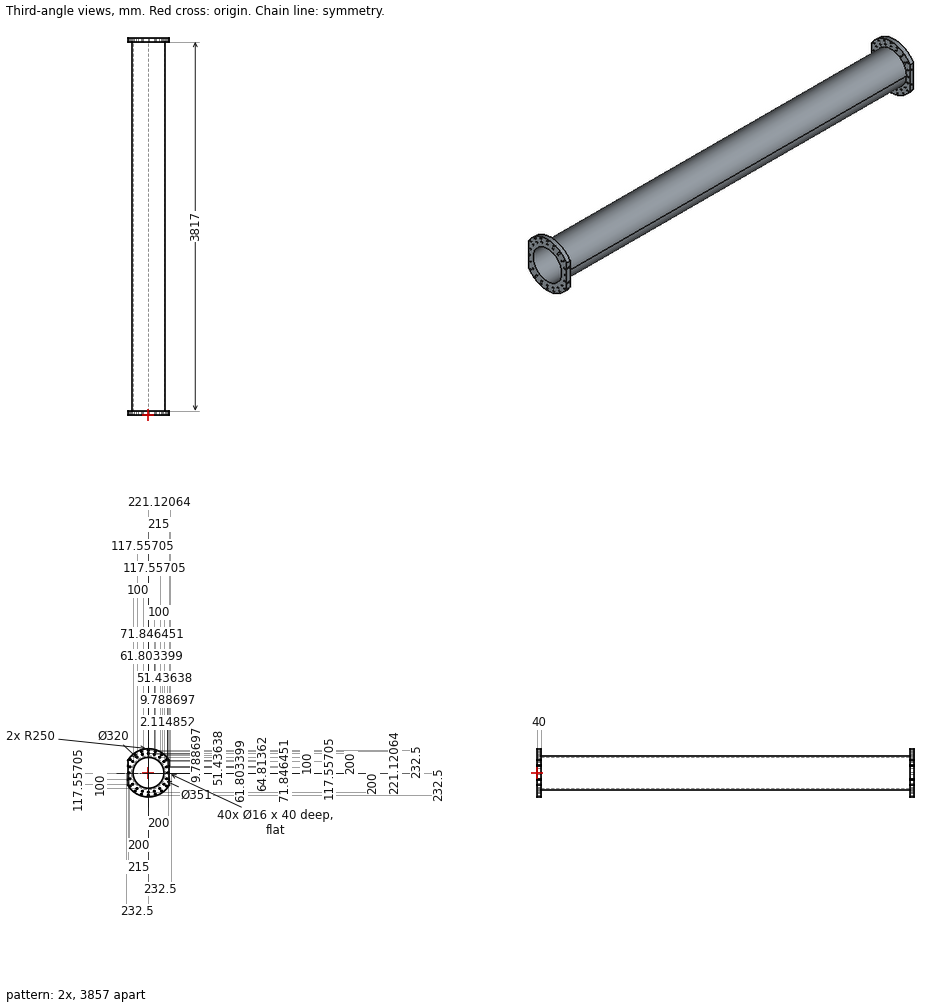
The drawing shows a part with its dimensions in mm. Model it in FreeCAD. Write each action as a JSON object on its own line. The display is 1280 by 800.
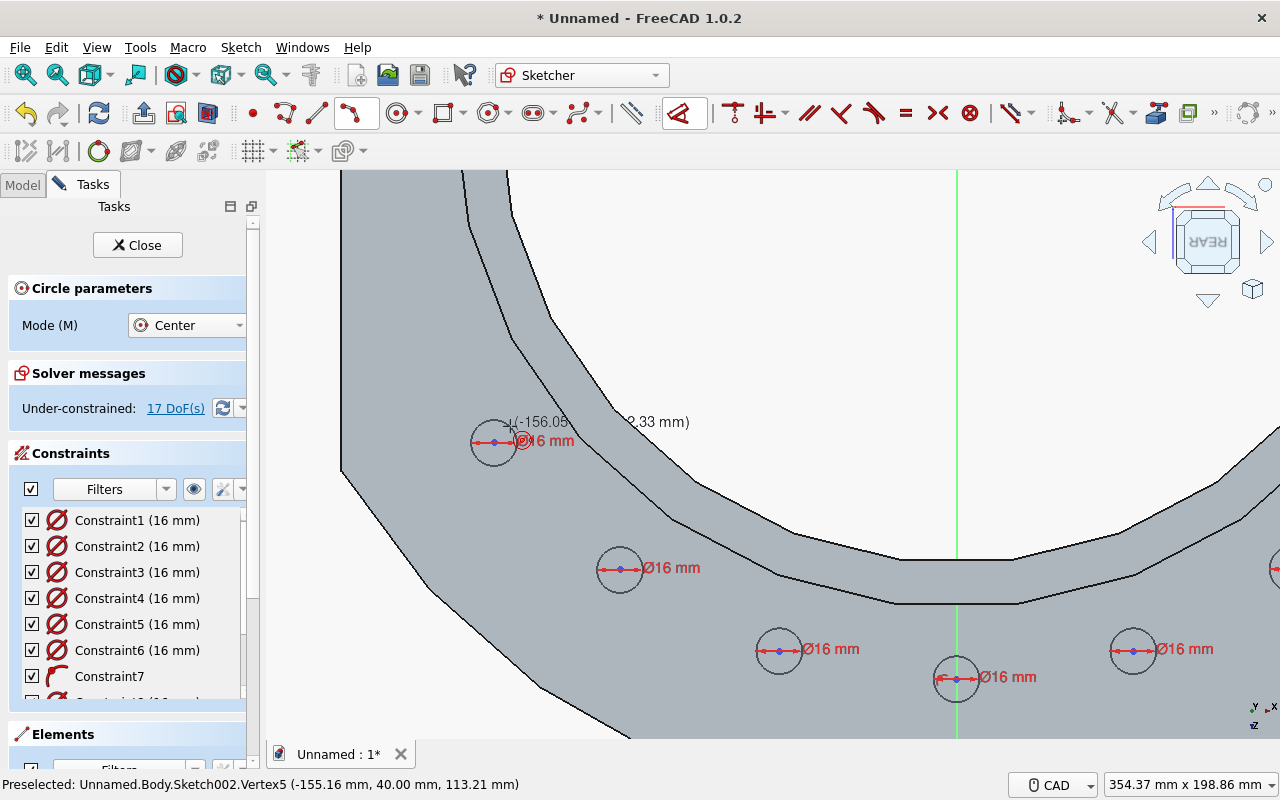
{"action": "left_click", "coordinate": [412, 282]}
{"action": "mouse_move", "coordinate": [428, 266]}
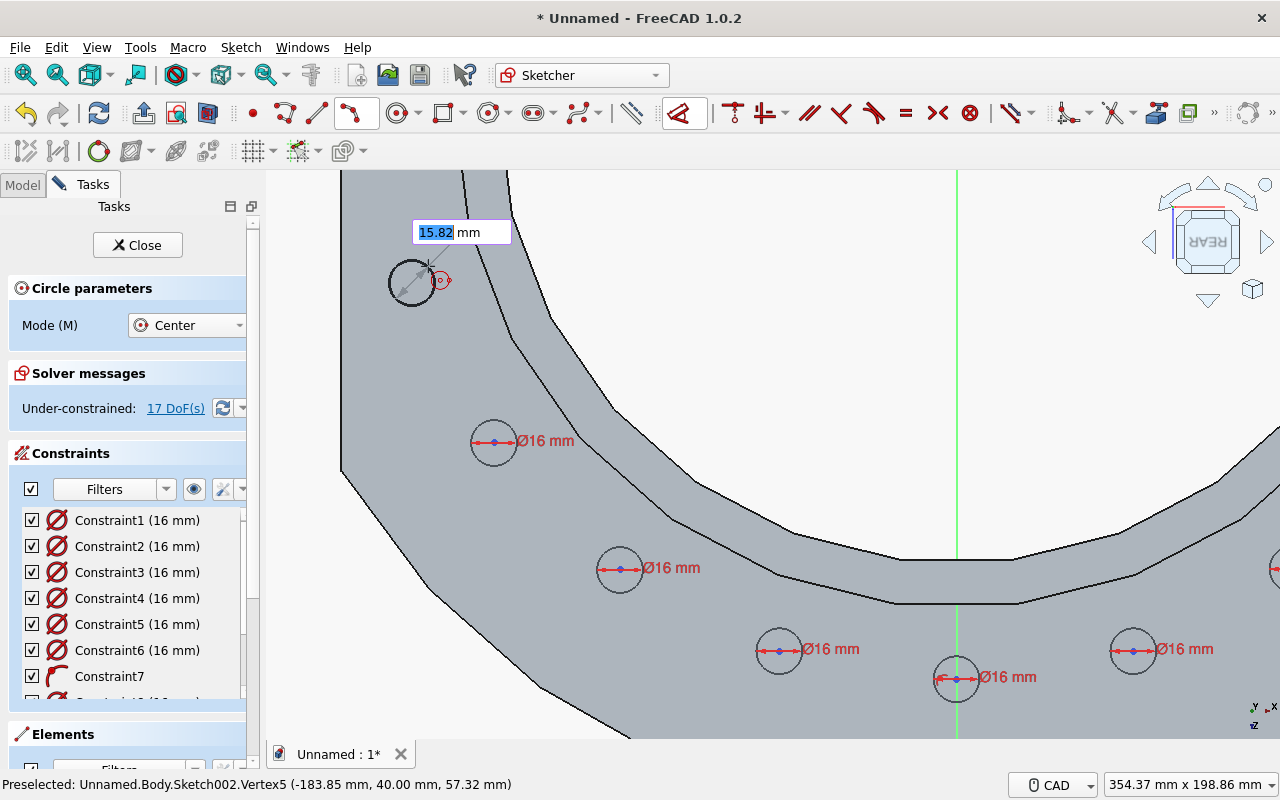
{"action": "type", "text": "16"}
{"action": "key", "text": "Return"}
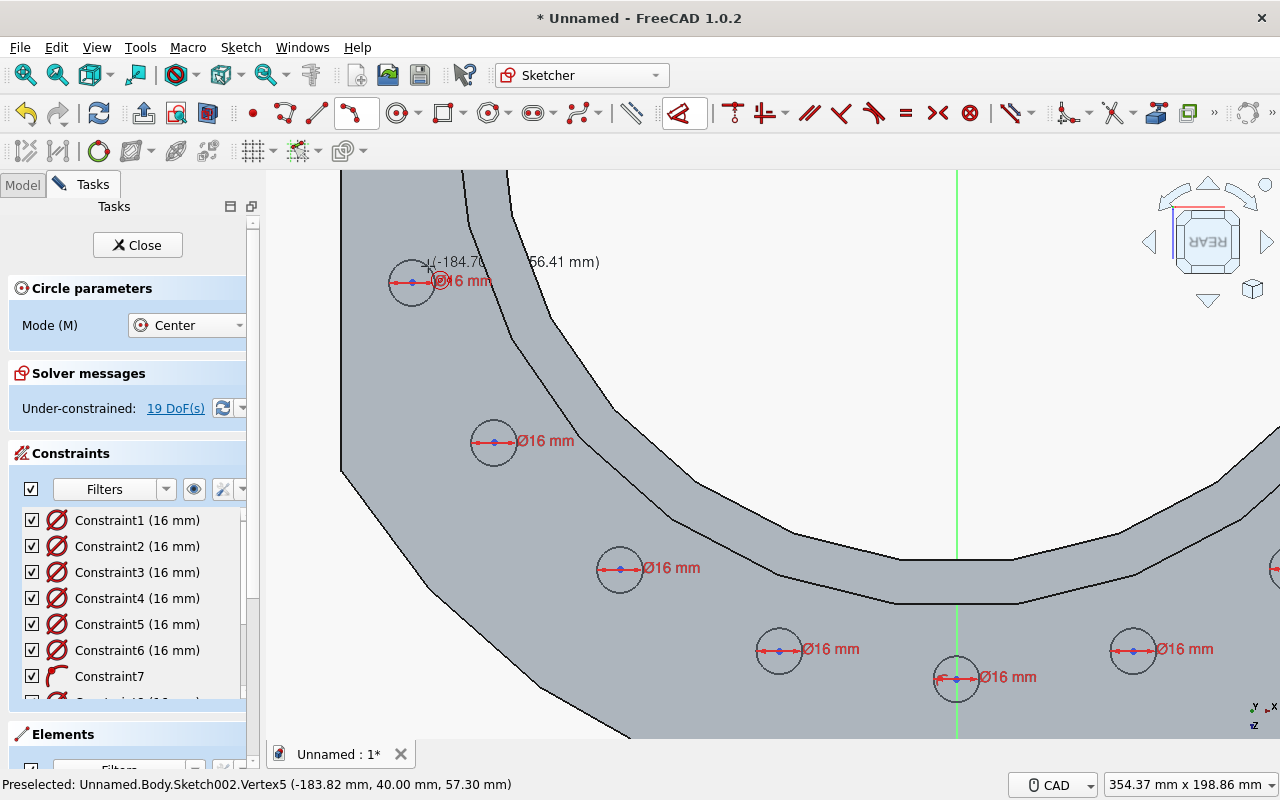
{"action": "scroll", "coordinate": [622, 569], "scroll_direction": "down", "scroll_amount": 7}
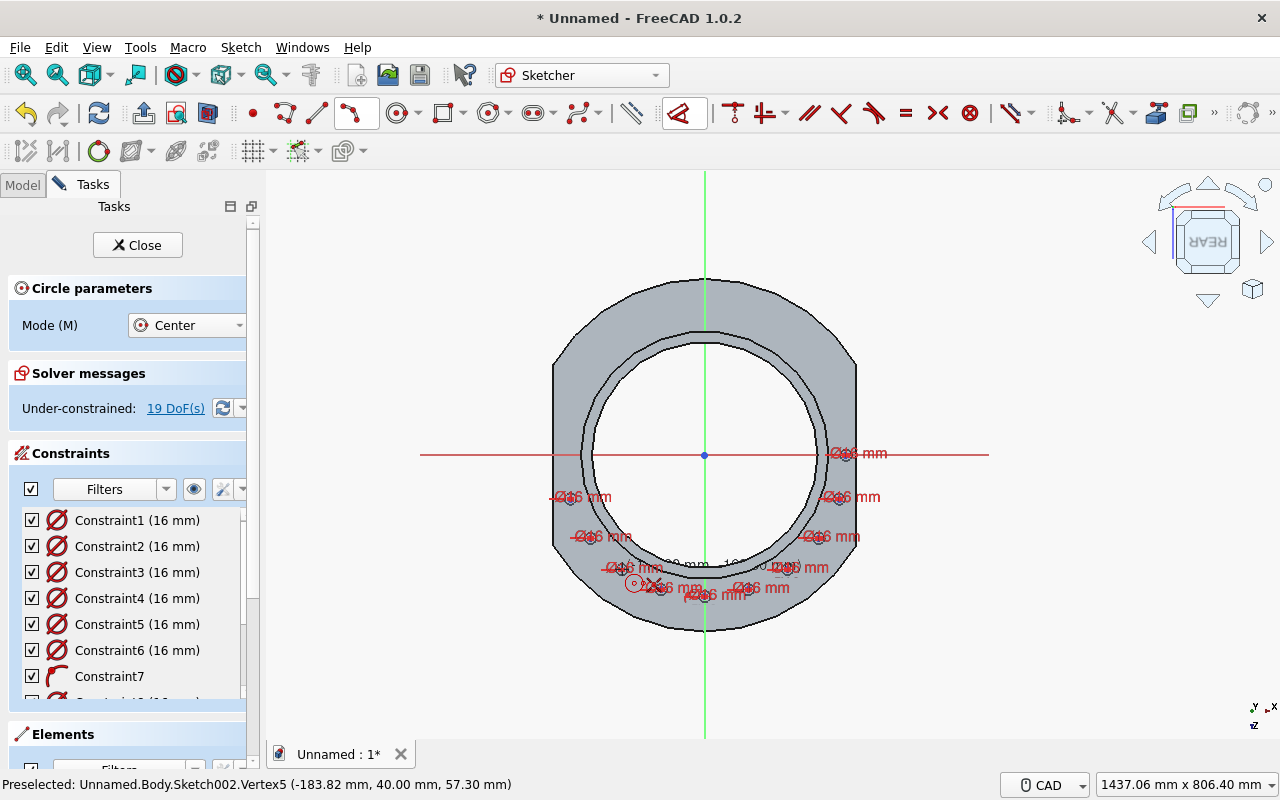
{"action": "scroll", "coordinate": [564, 455], "scroll_direction": "up", "scroll_amount": 7}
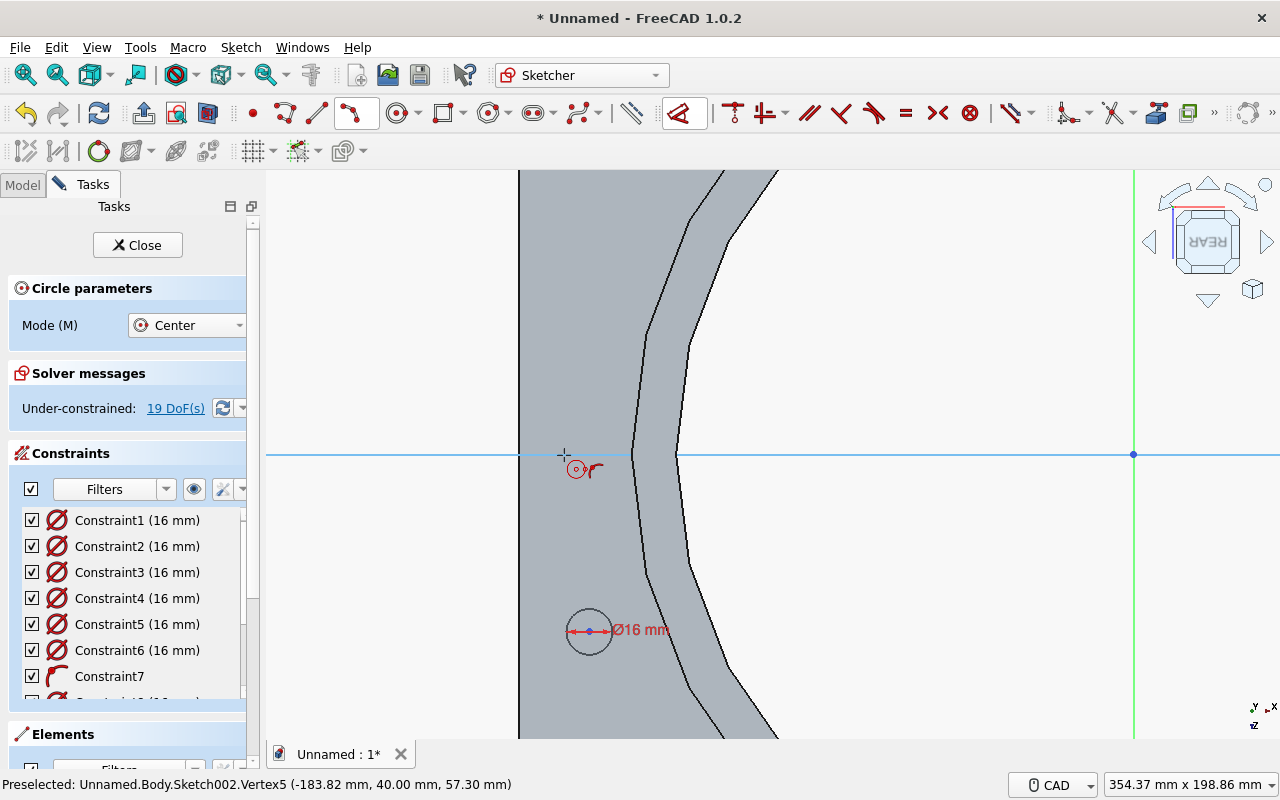
{"action": "left_click", "coordinate": [562, 455]}
{"action": "mouse_move", "coordinate": [578, 438]}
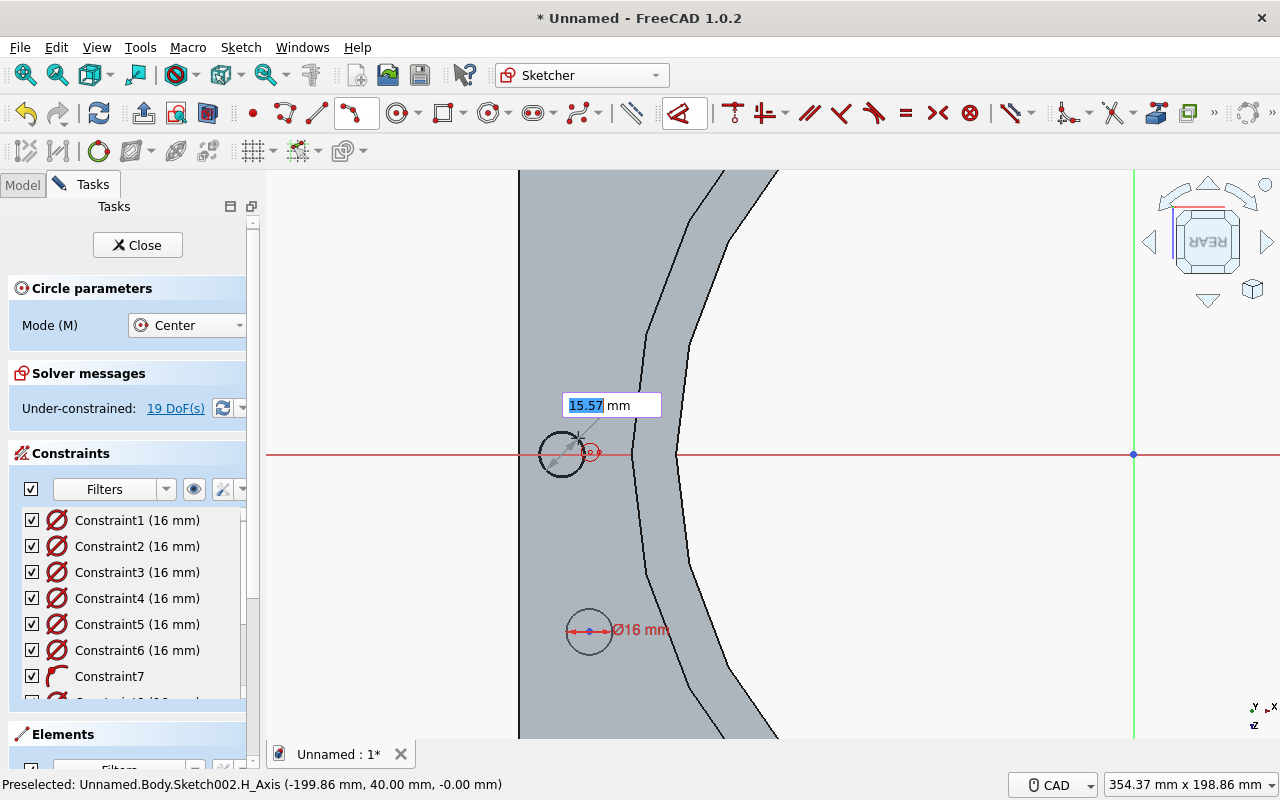
{"action": "type", "text": "16"}
{"action": "key", "text": "Return"}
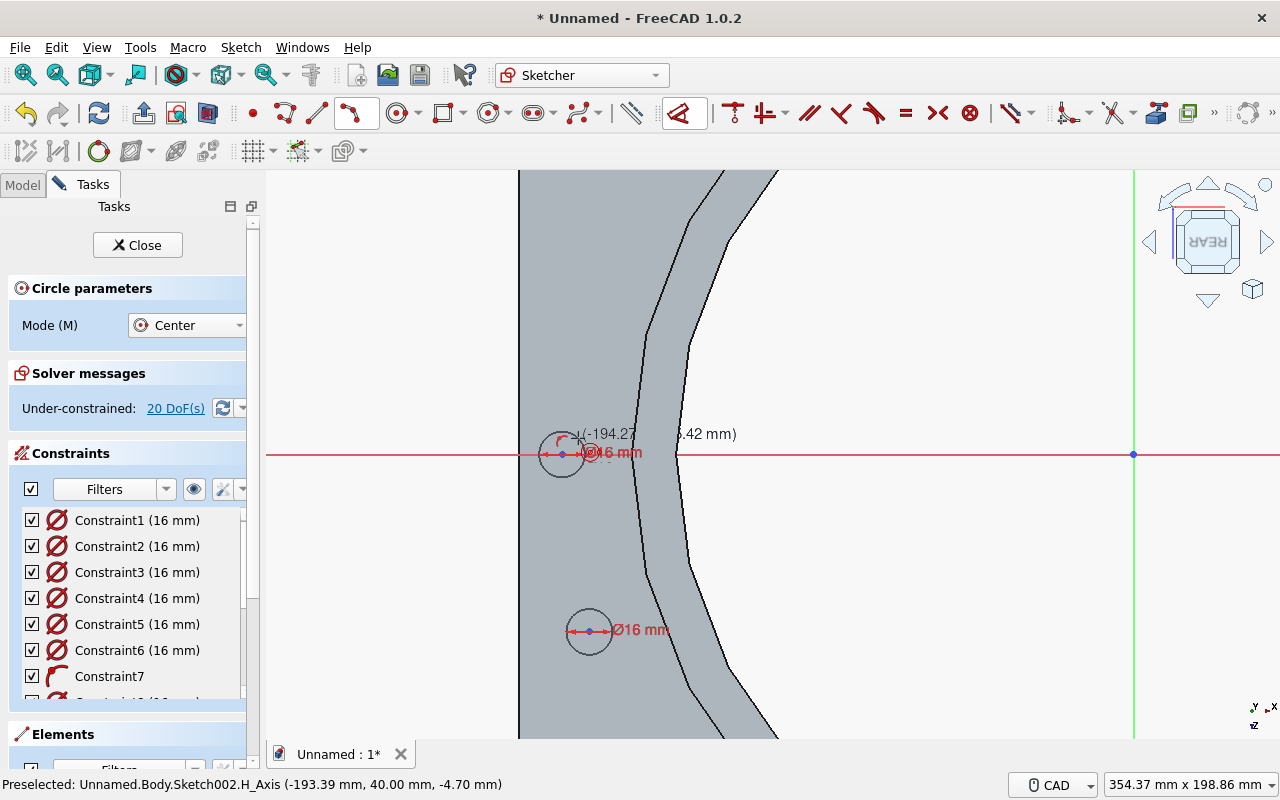
{"action": "left_click", "coordinate": [590, 278]}
{"action": "mouse_move", "coordinate": [606, 261]}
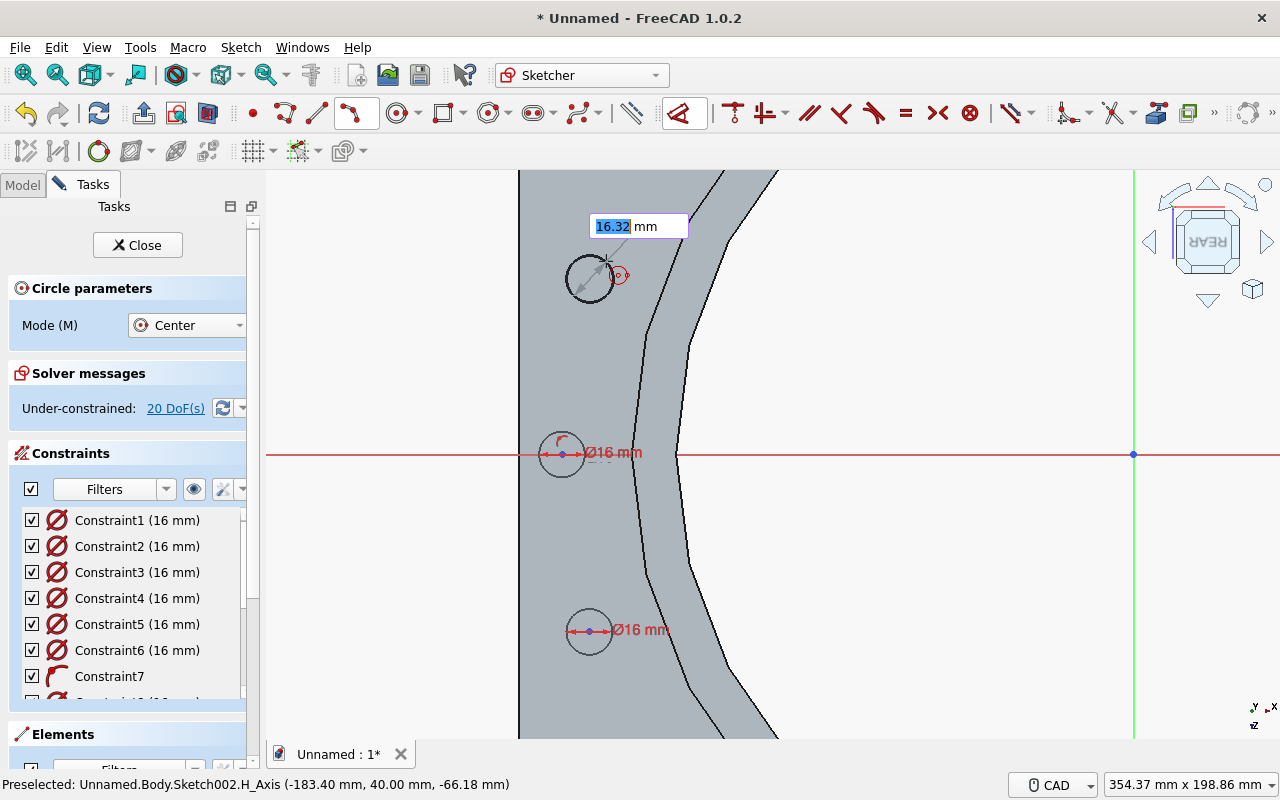
{"action": "type", "text": "16"}
{"action": "key", "text": "Return"}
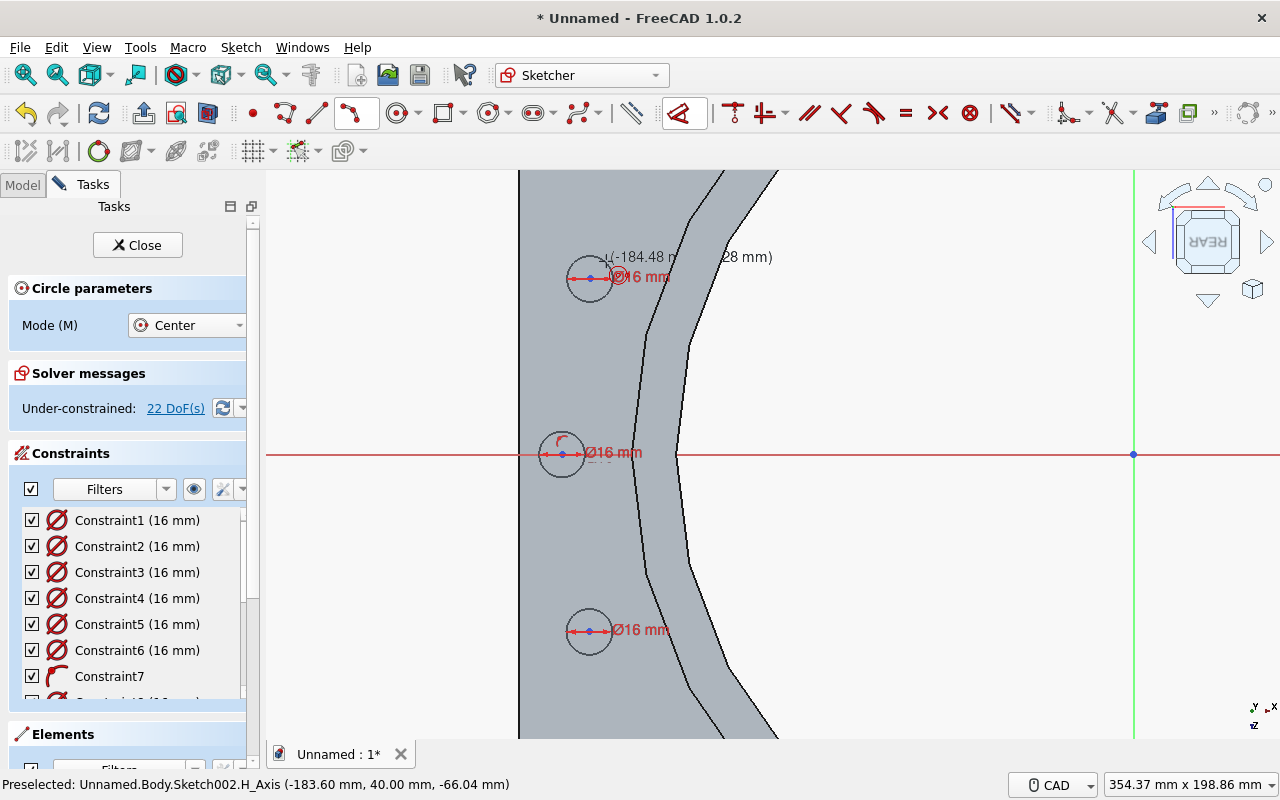
{"action": "scroll", "coordinate": [564, 454], "scroll_direction": "down", "scroll_amount": 7}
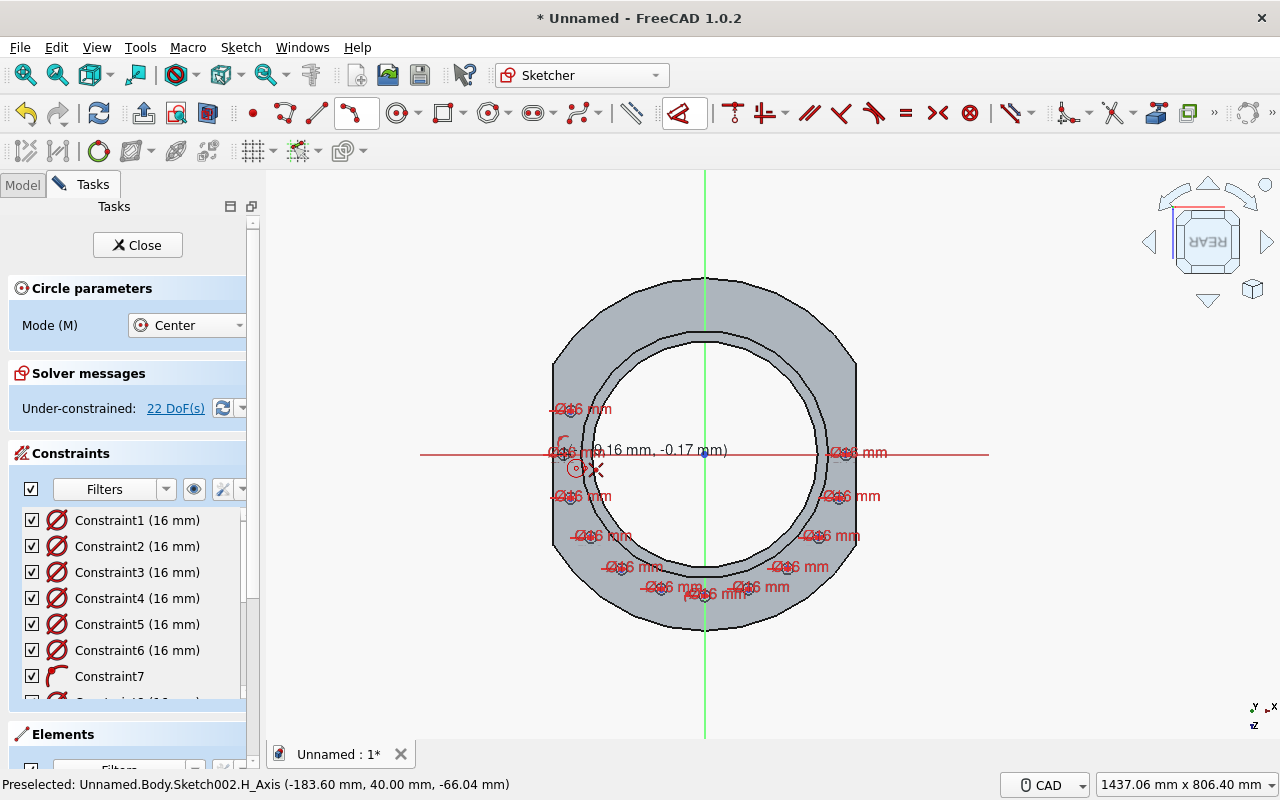
{"action": "scroll", "coordinate": [591, 372], "scroll_direction": "up", "scroll_amount": 7}